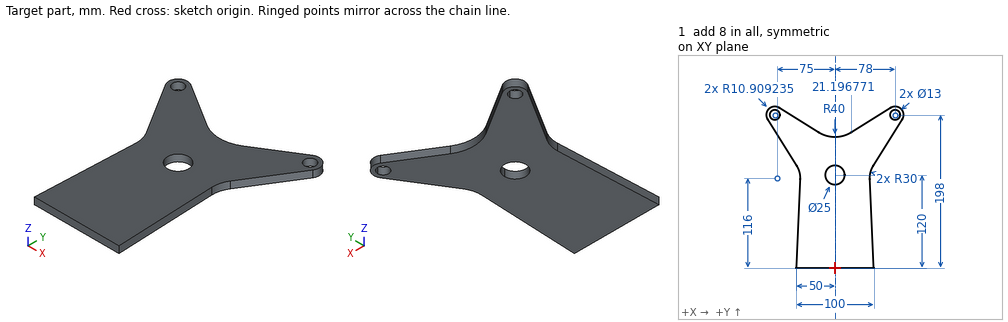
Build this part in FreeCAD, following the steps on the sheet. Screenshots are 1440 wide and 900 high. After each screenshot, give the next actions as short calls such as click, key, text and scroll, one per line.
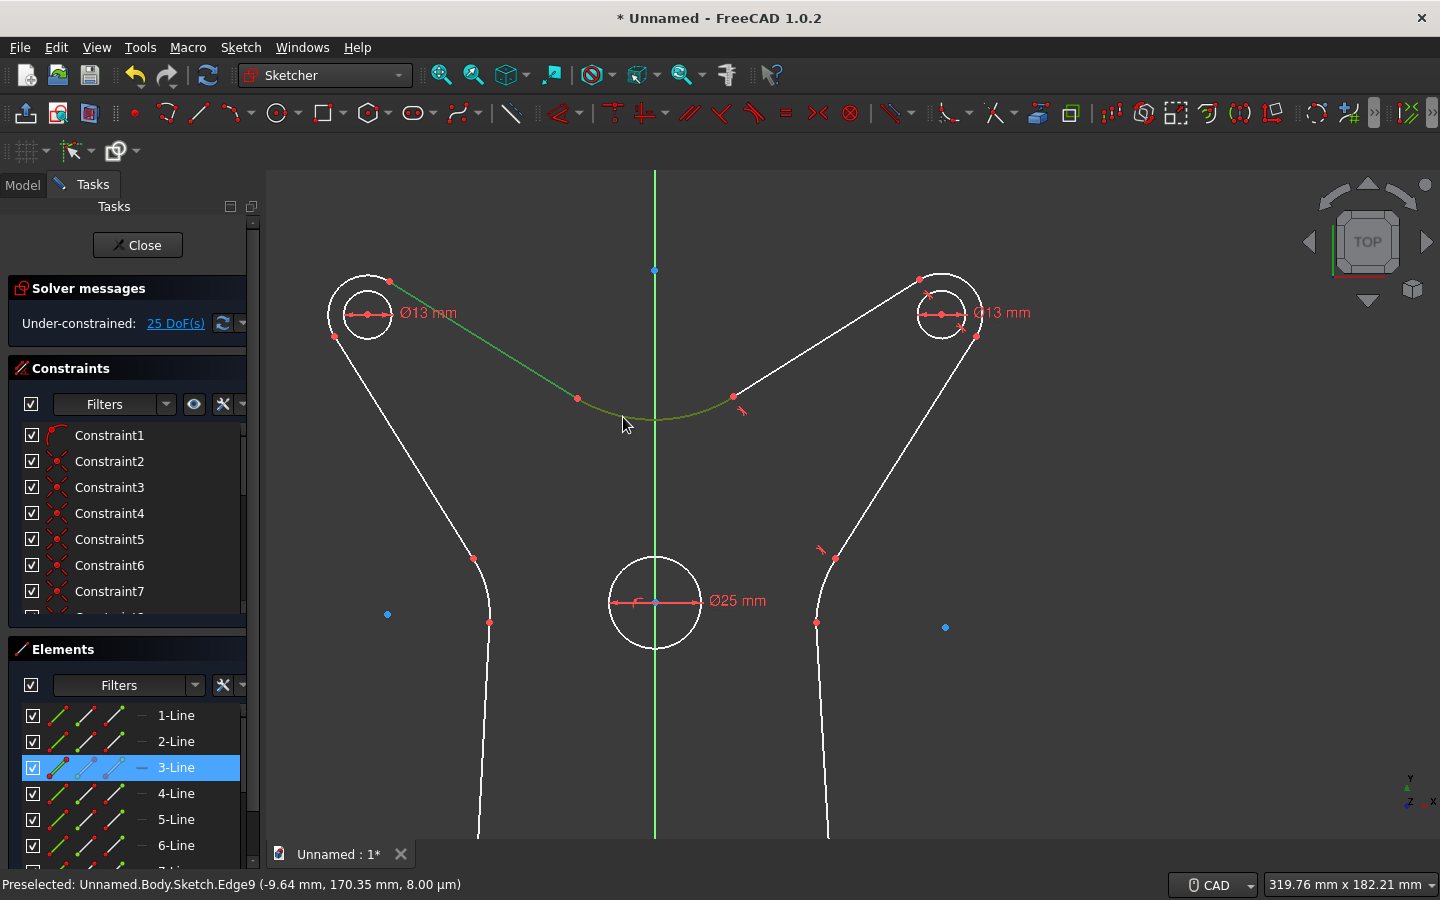
key(t)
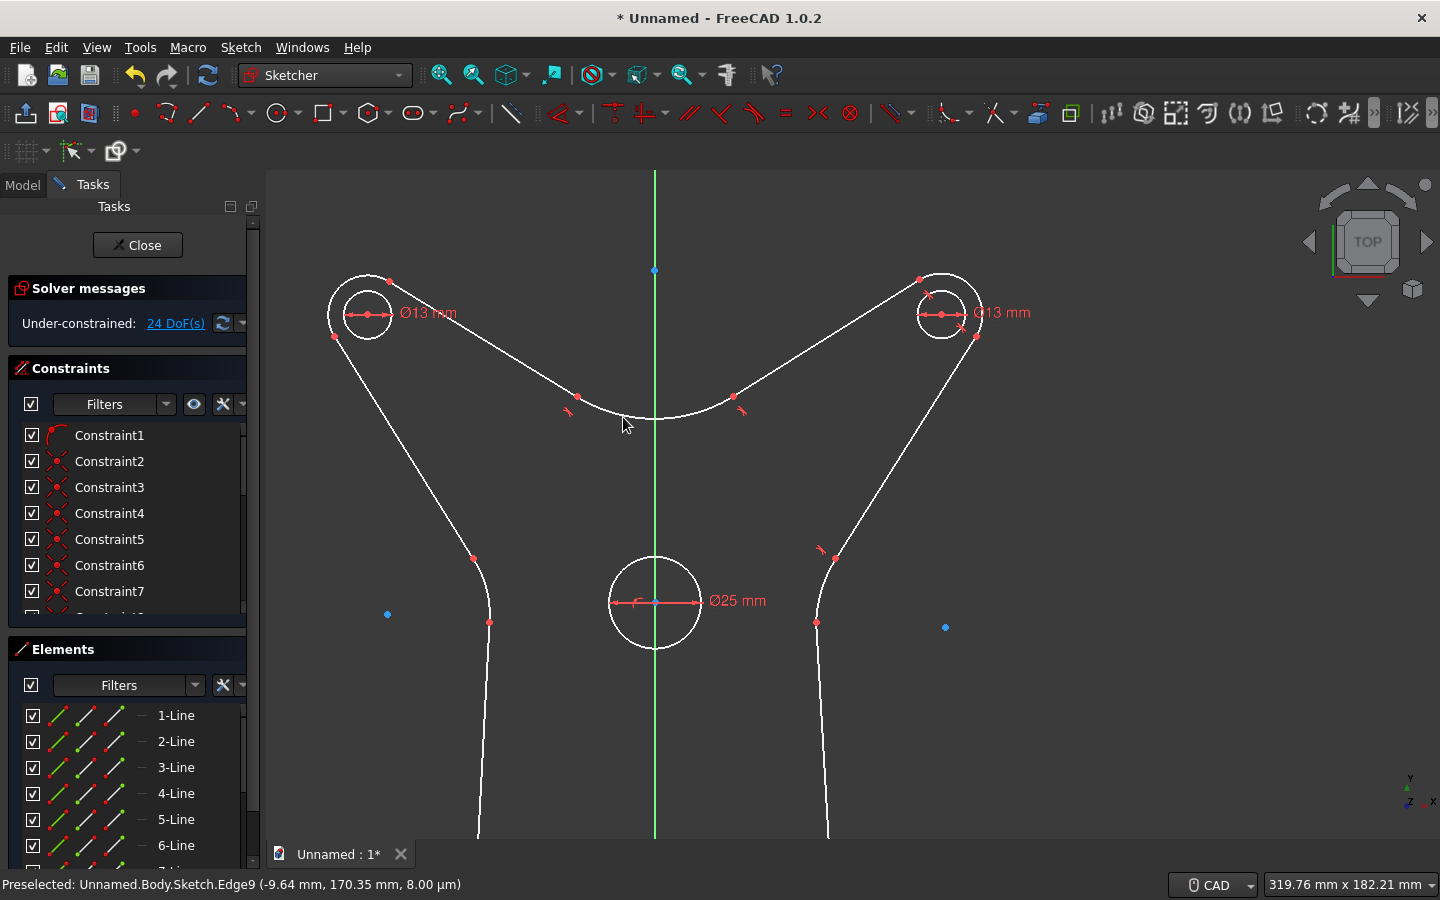
click(521, 362)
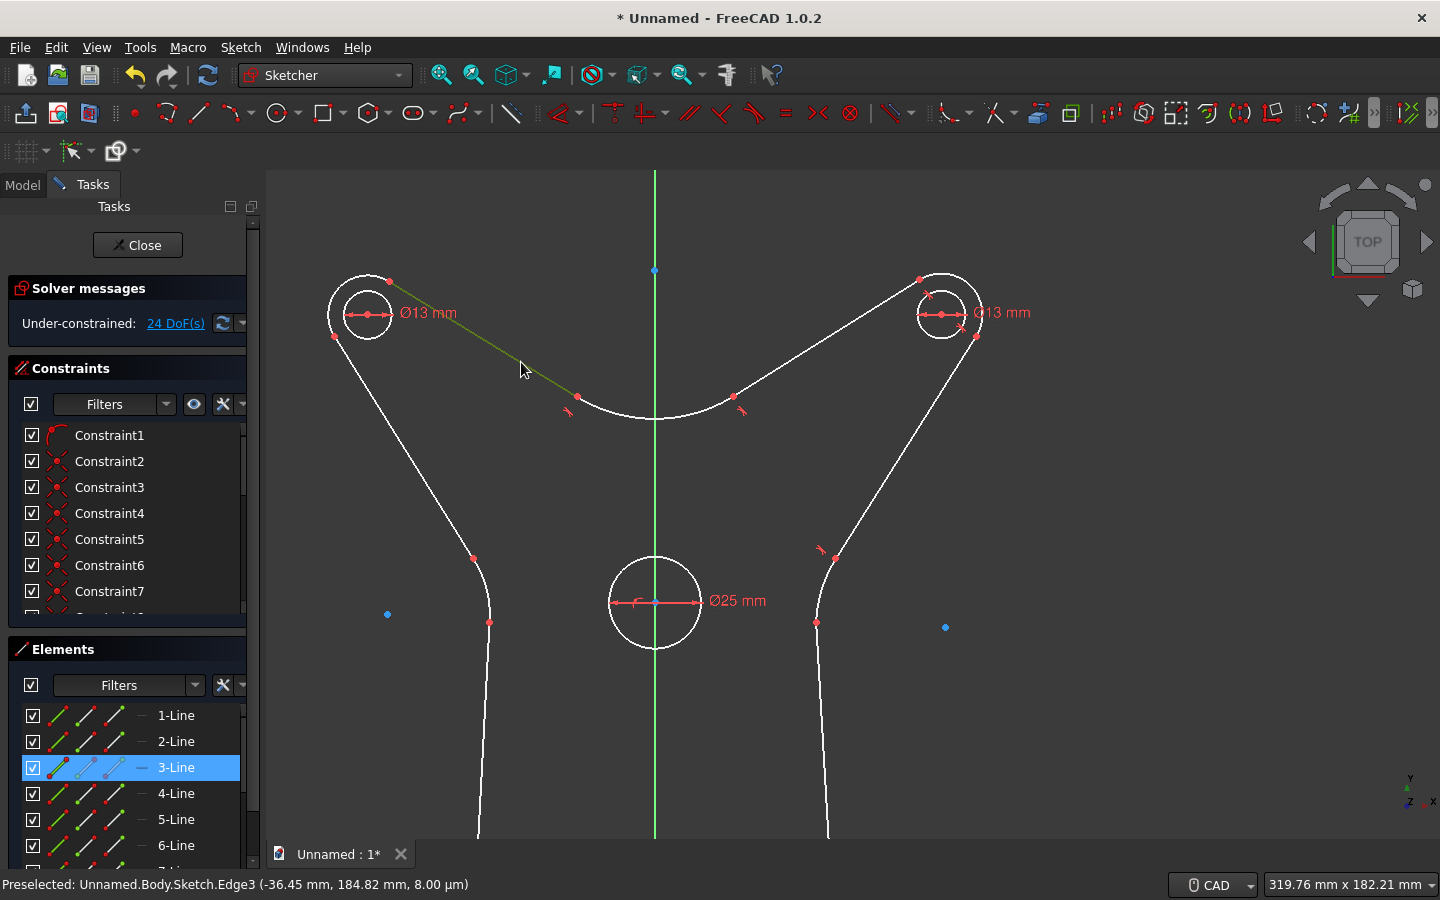
click(358, 277)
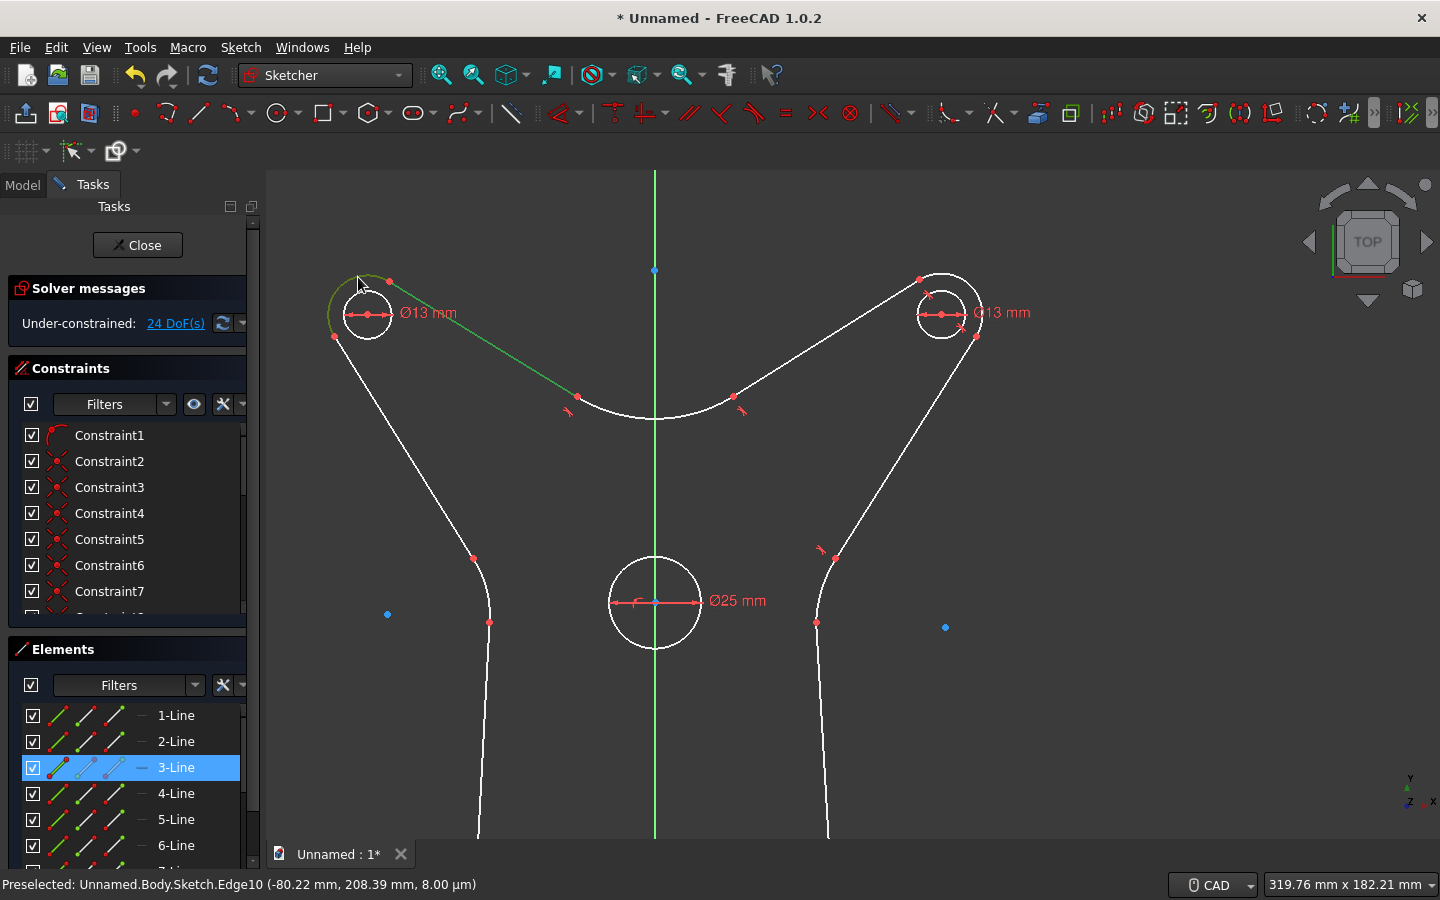
click(754, 114)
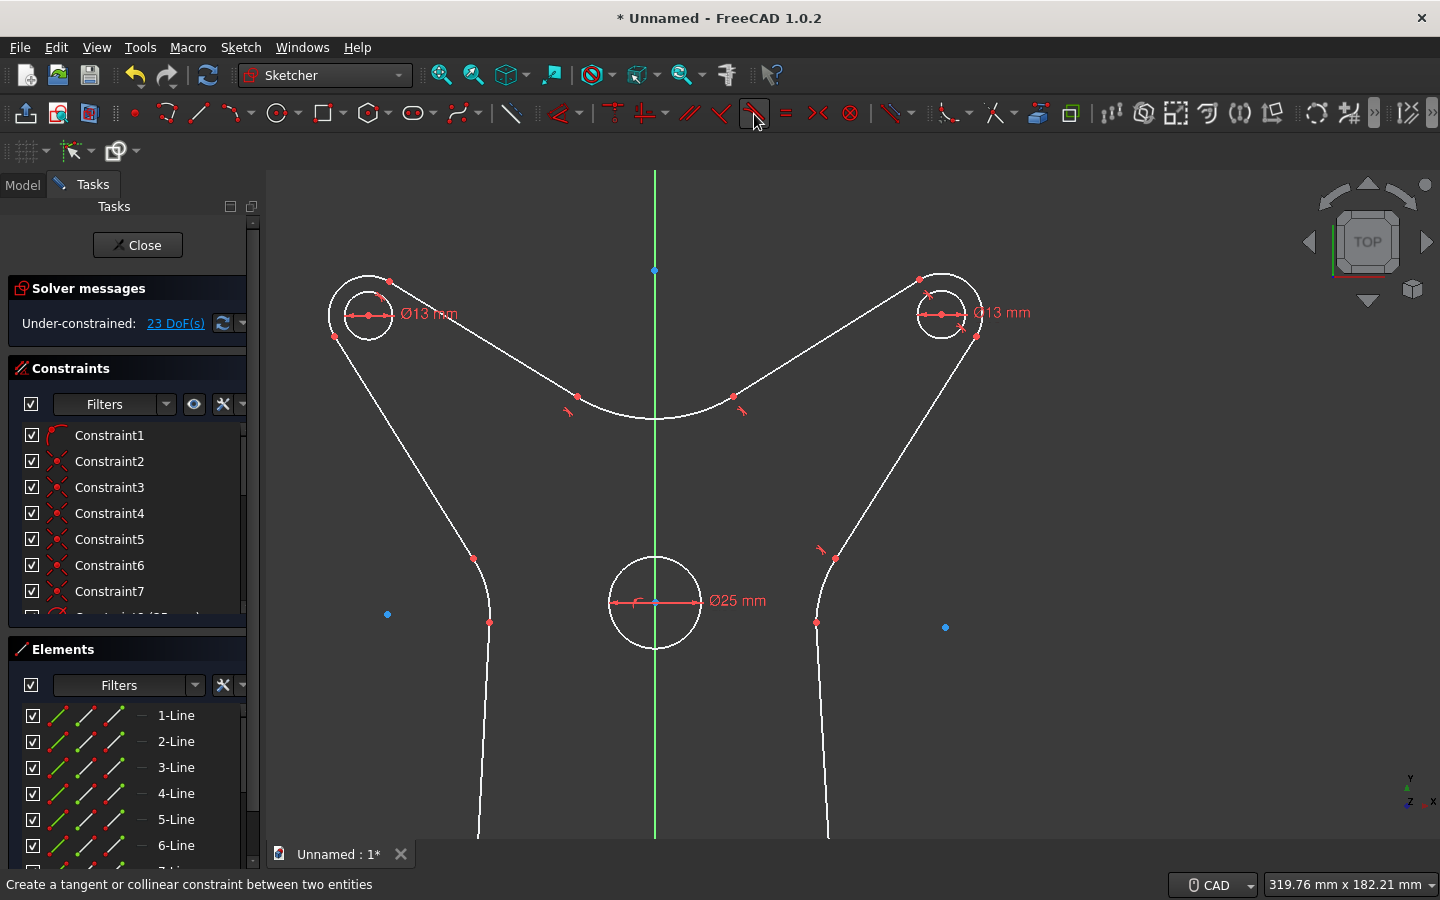
click(376, 403)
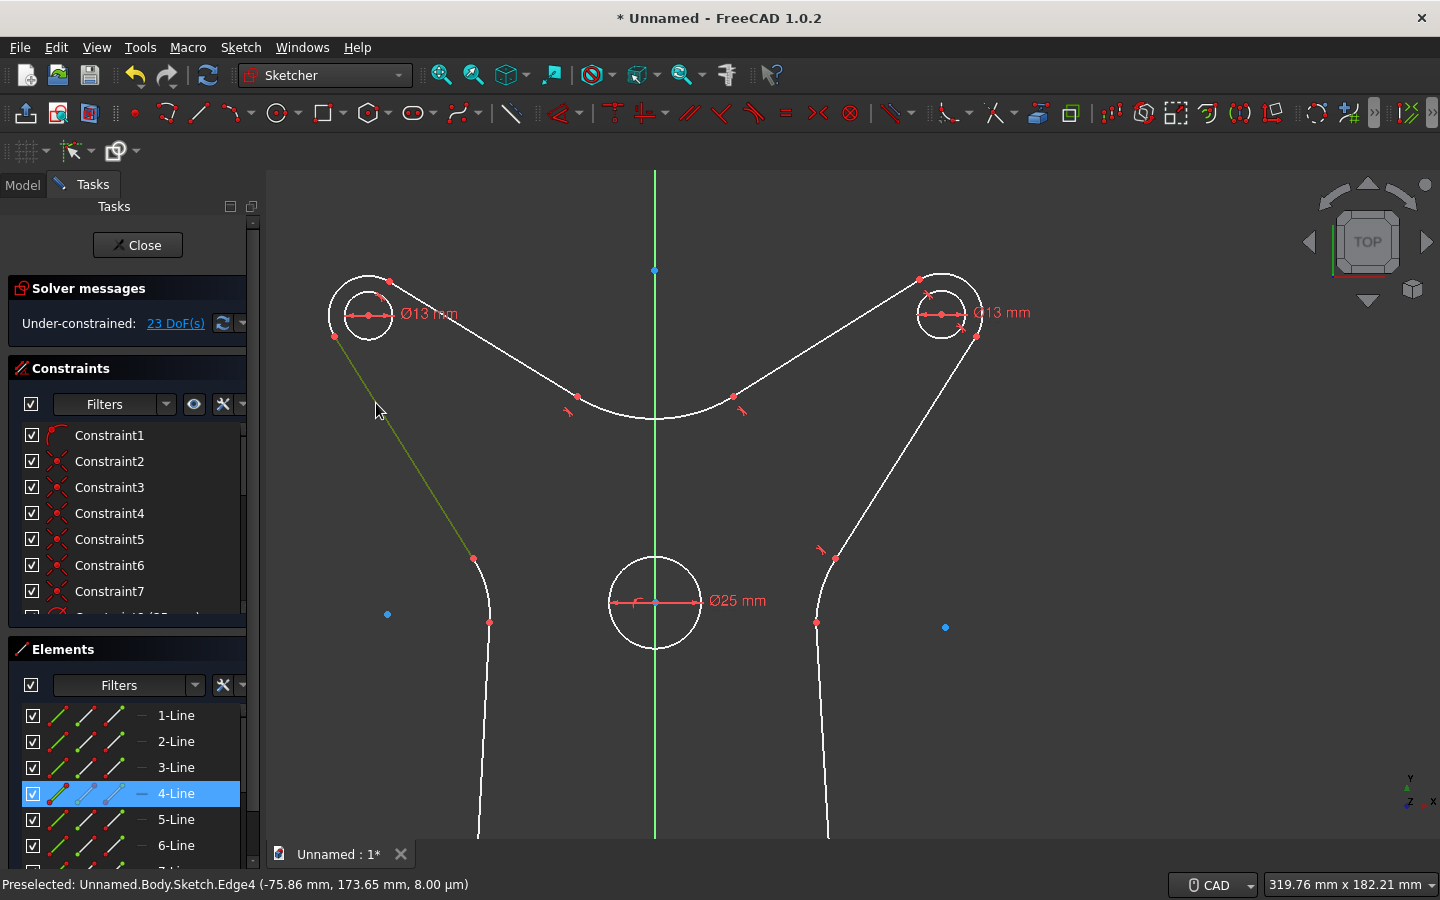
click(359, 277)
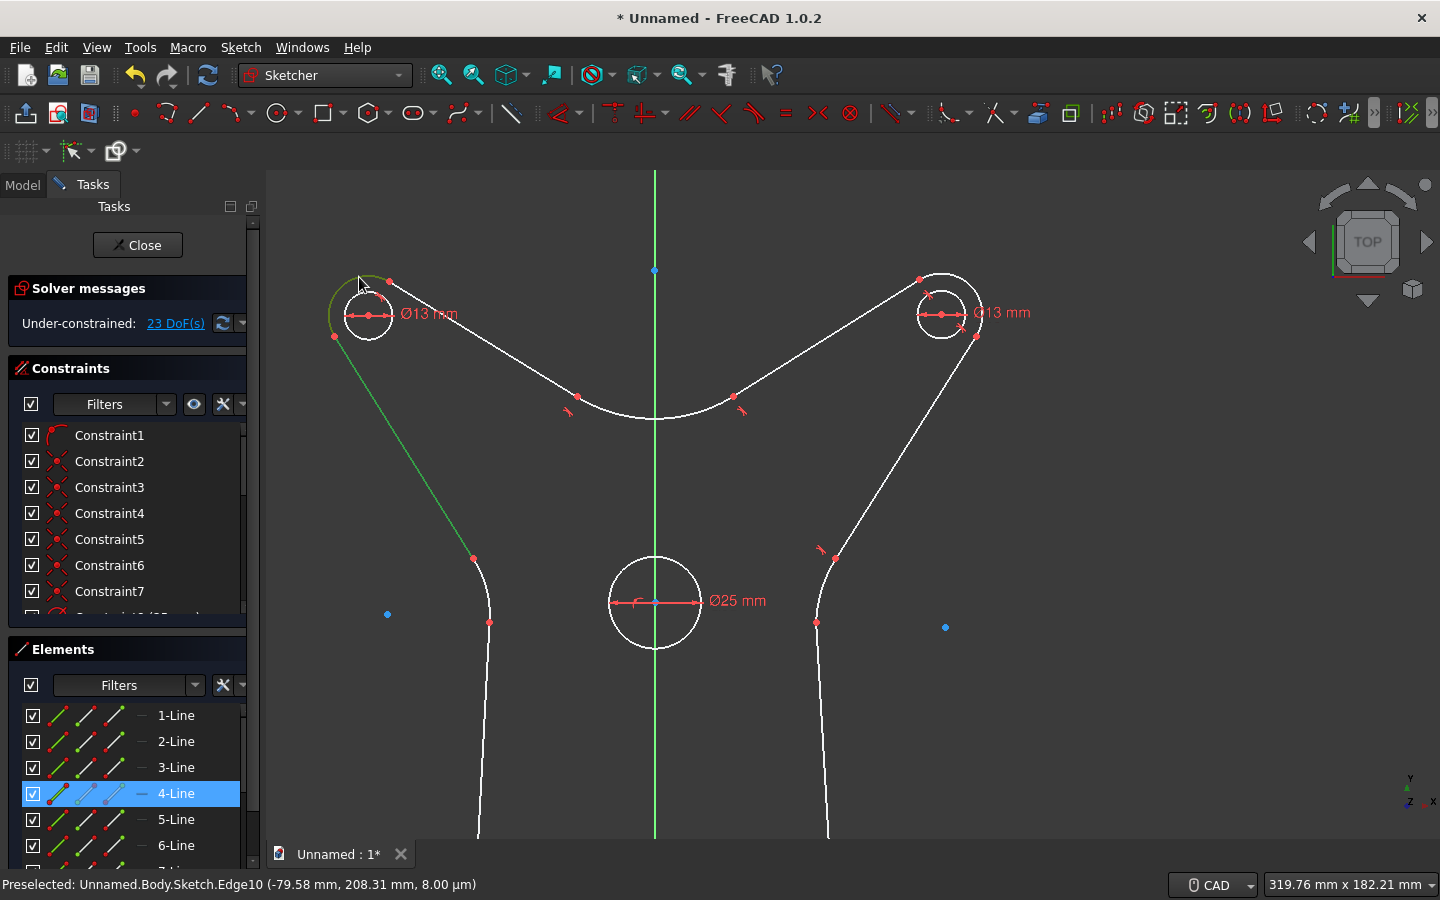
click(754, 114)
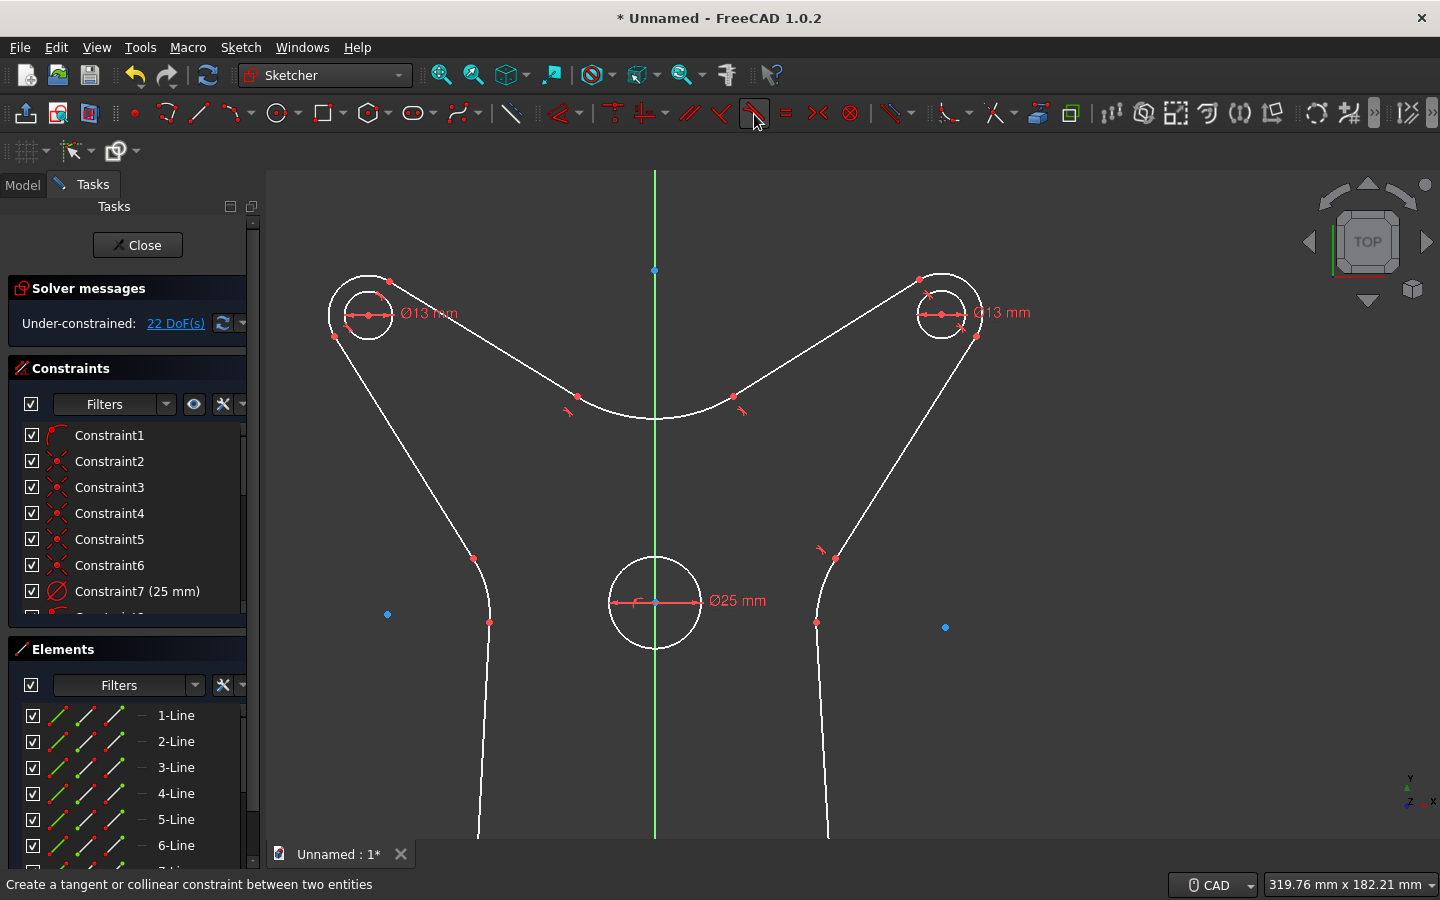
click(376, 403)